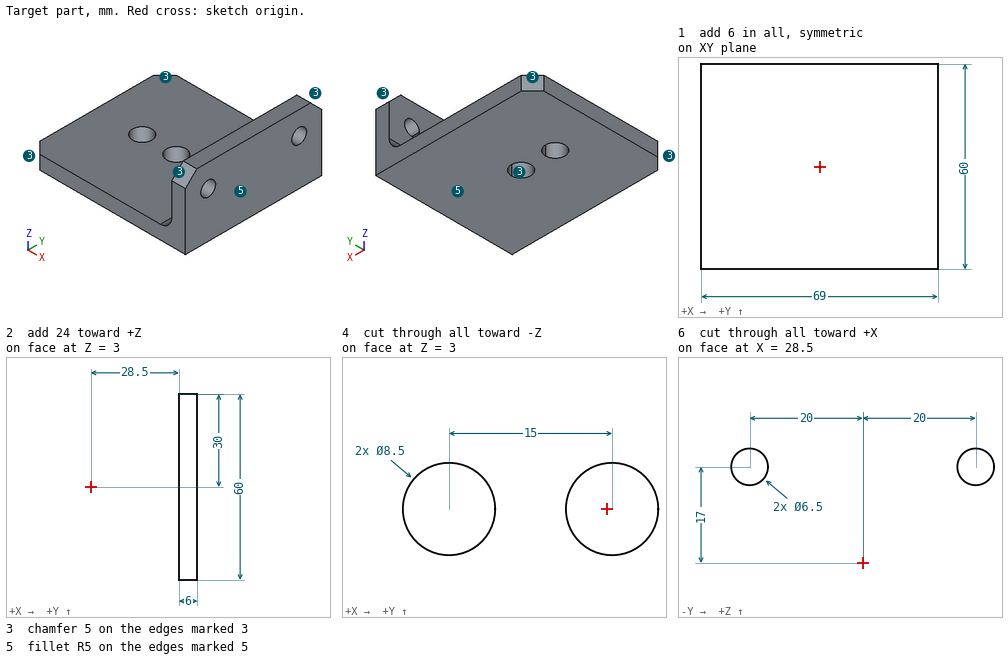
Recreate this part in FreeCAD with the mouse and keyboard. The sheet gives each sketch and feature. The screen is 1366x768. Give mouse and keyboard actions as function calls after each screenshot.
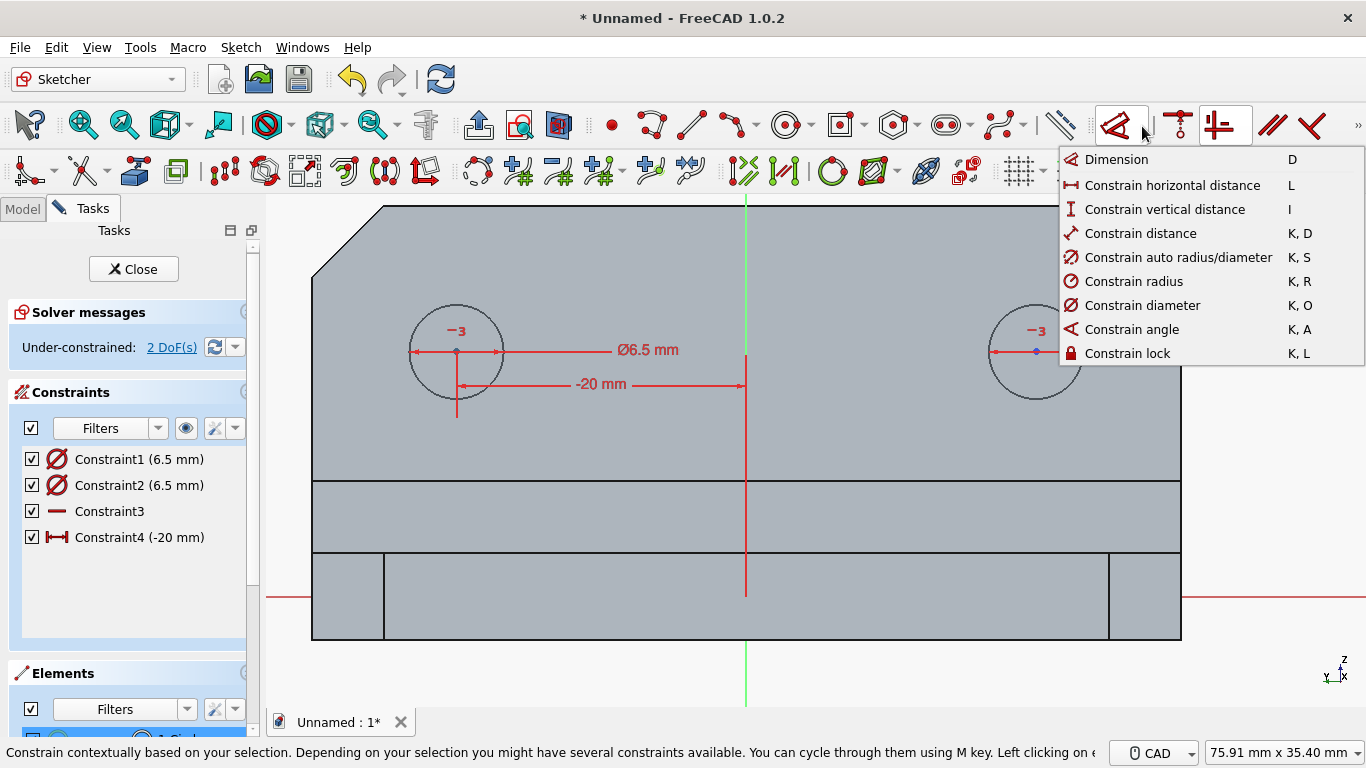
click(1212, 209)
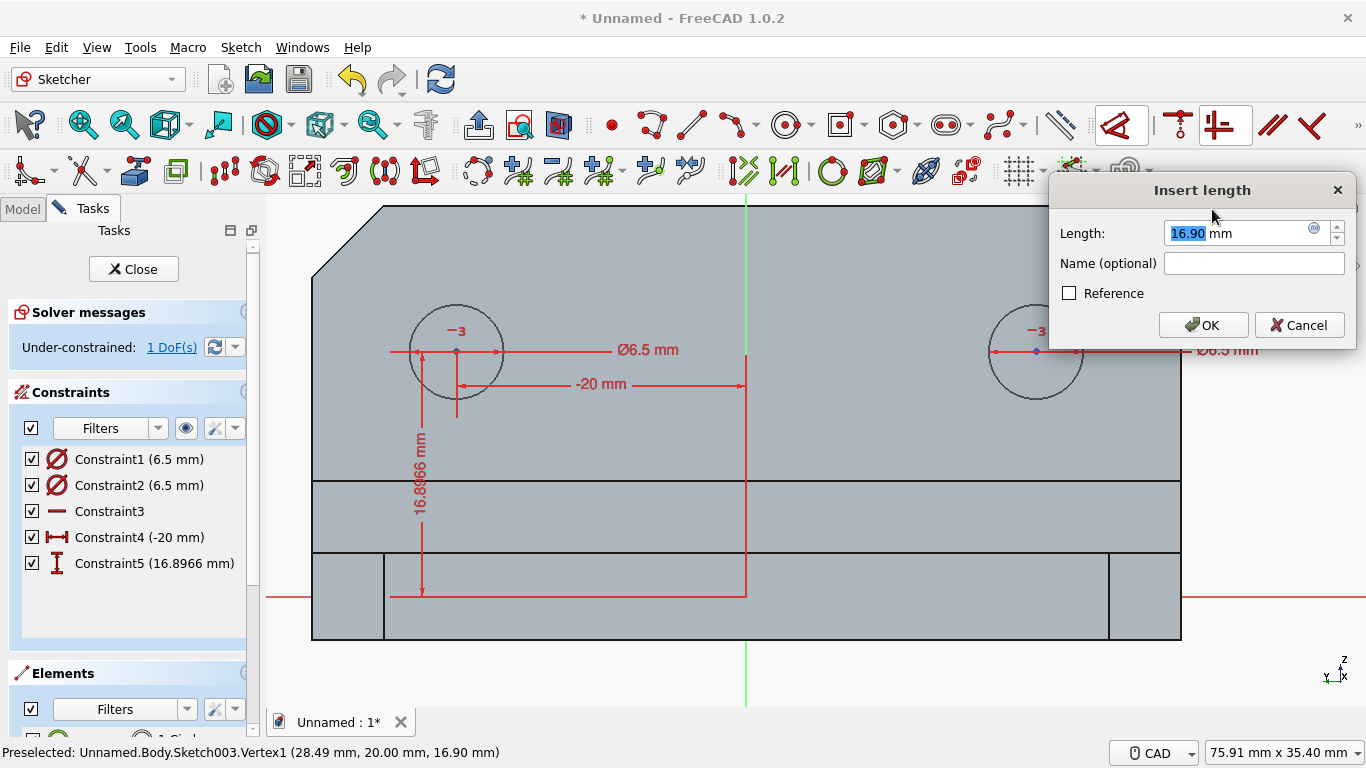
text(17)
key(Return)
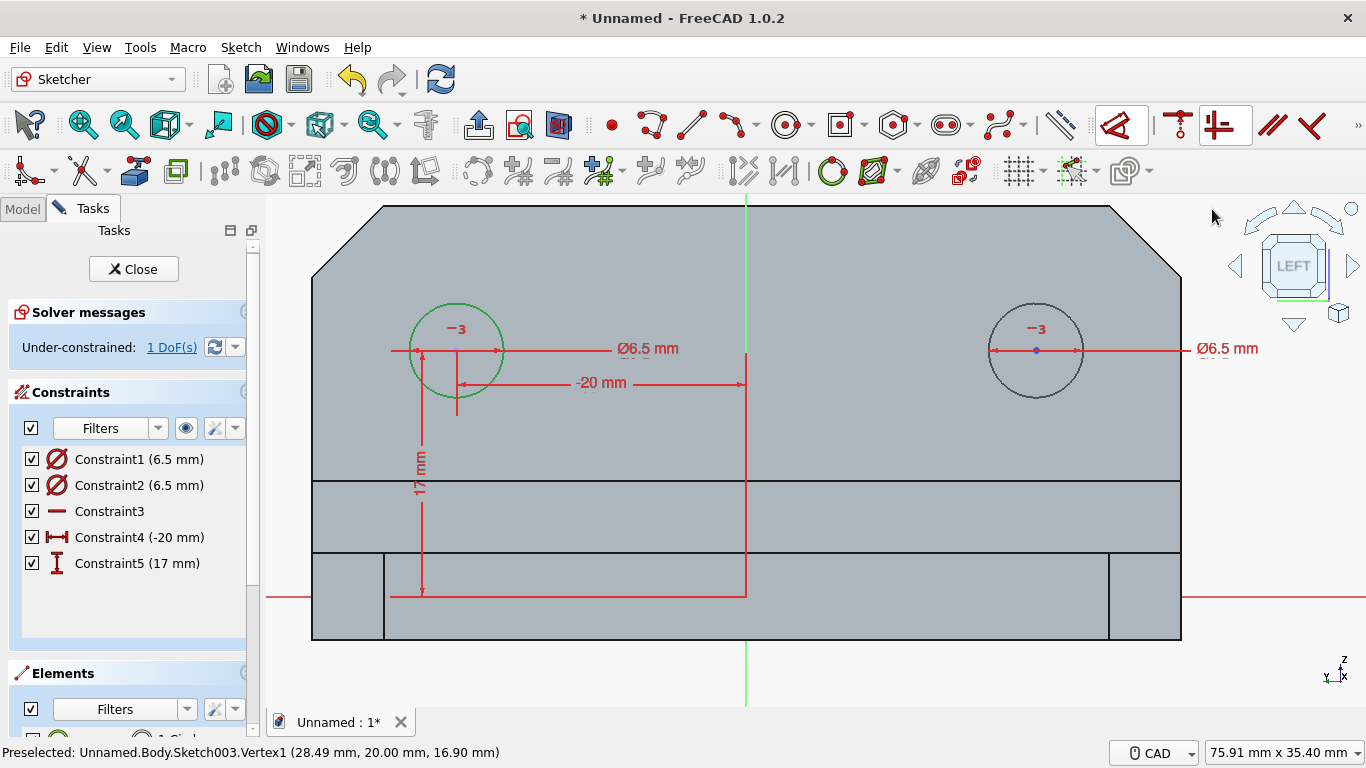
click(1036, 351)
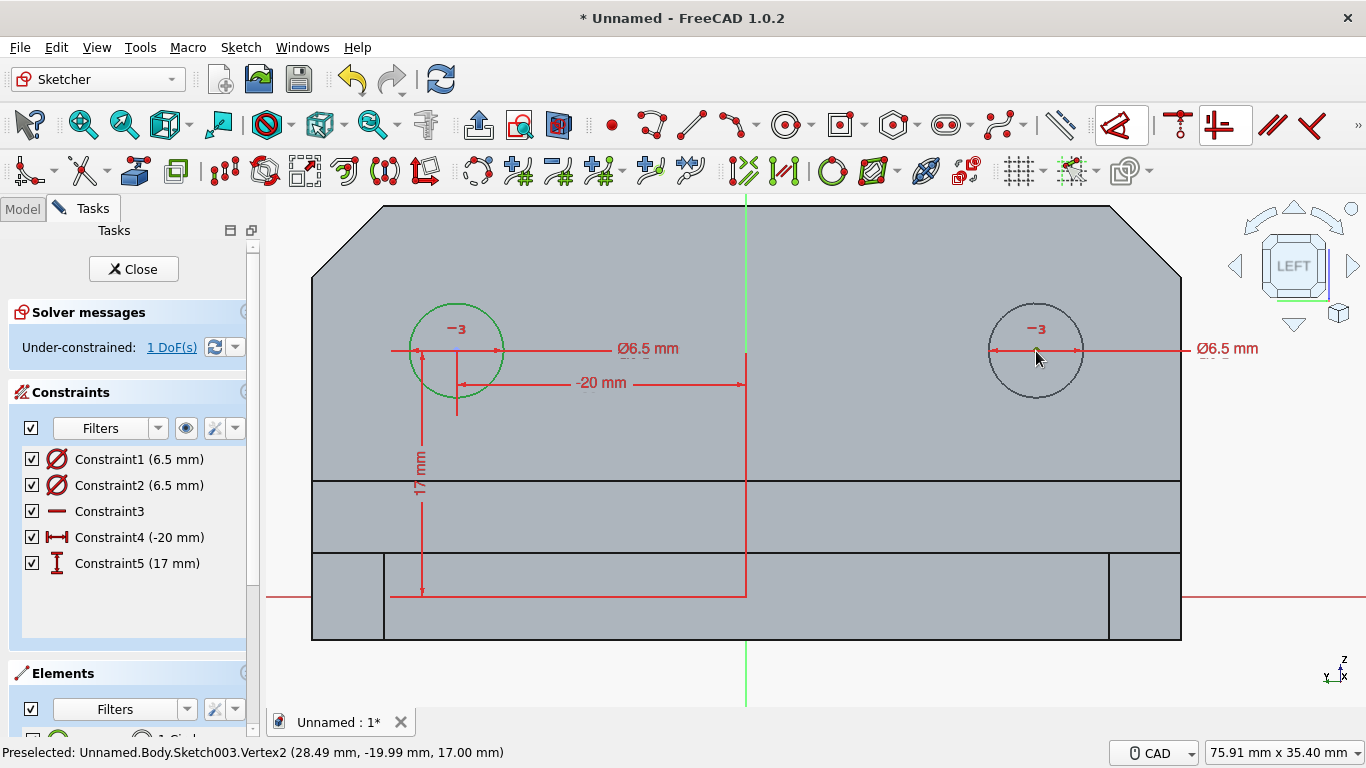
key(l)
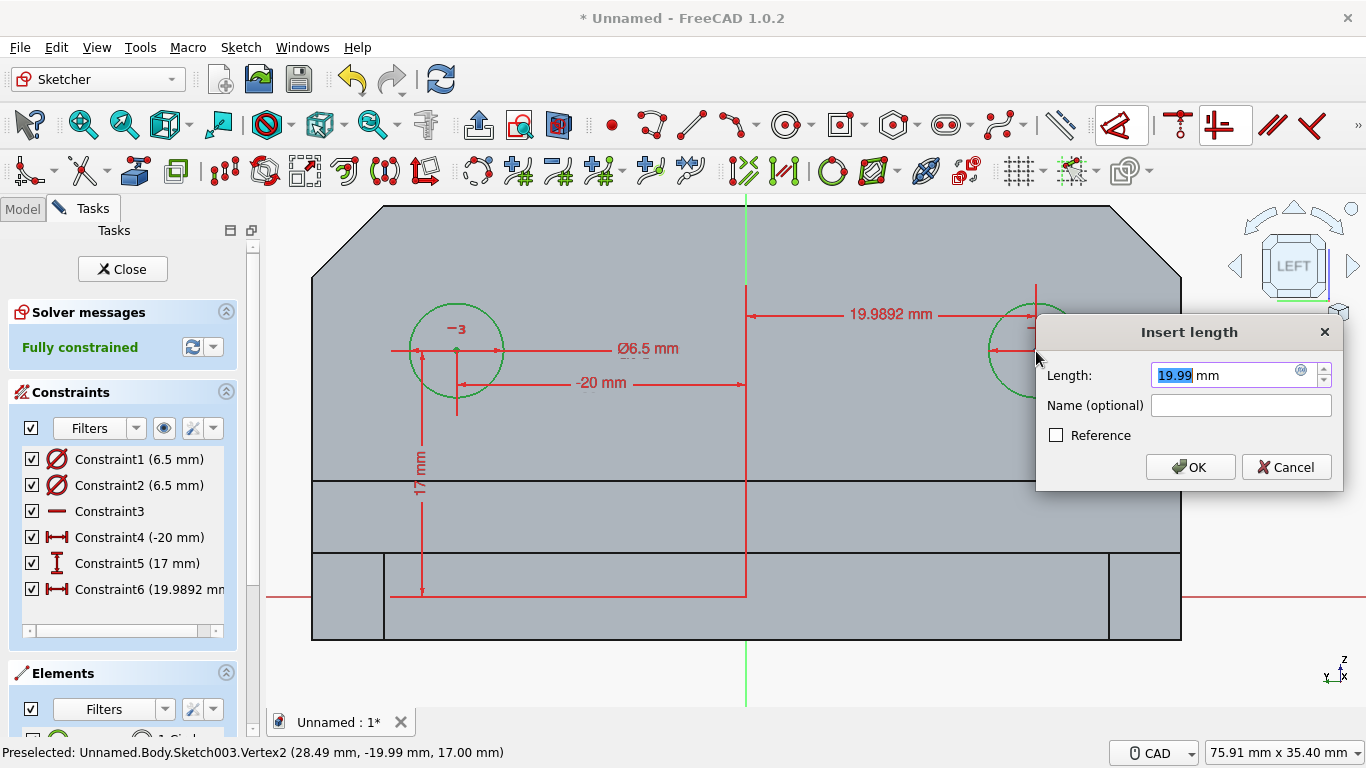
text(20)
key(Return)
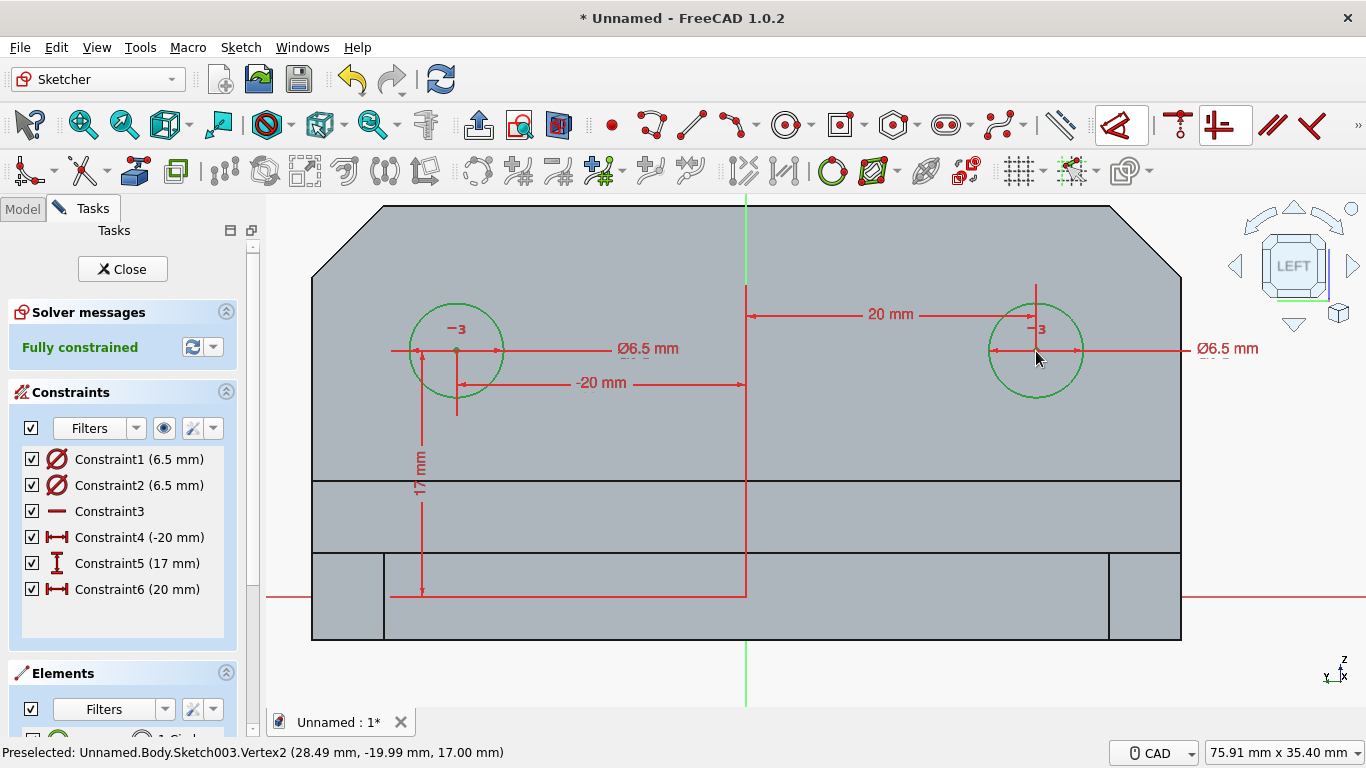
click(123, 269)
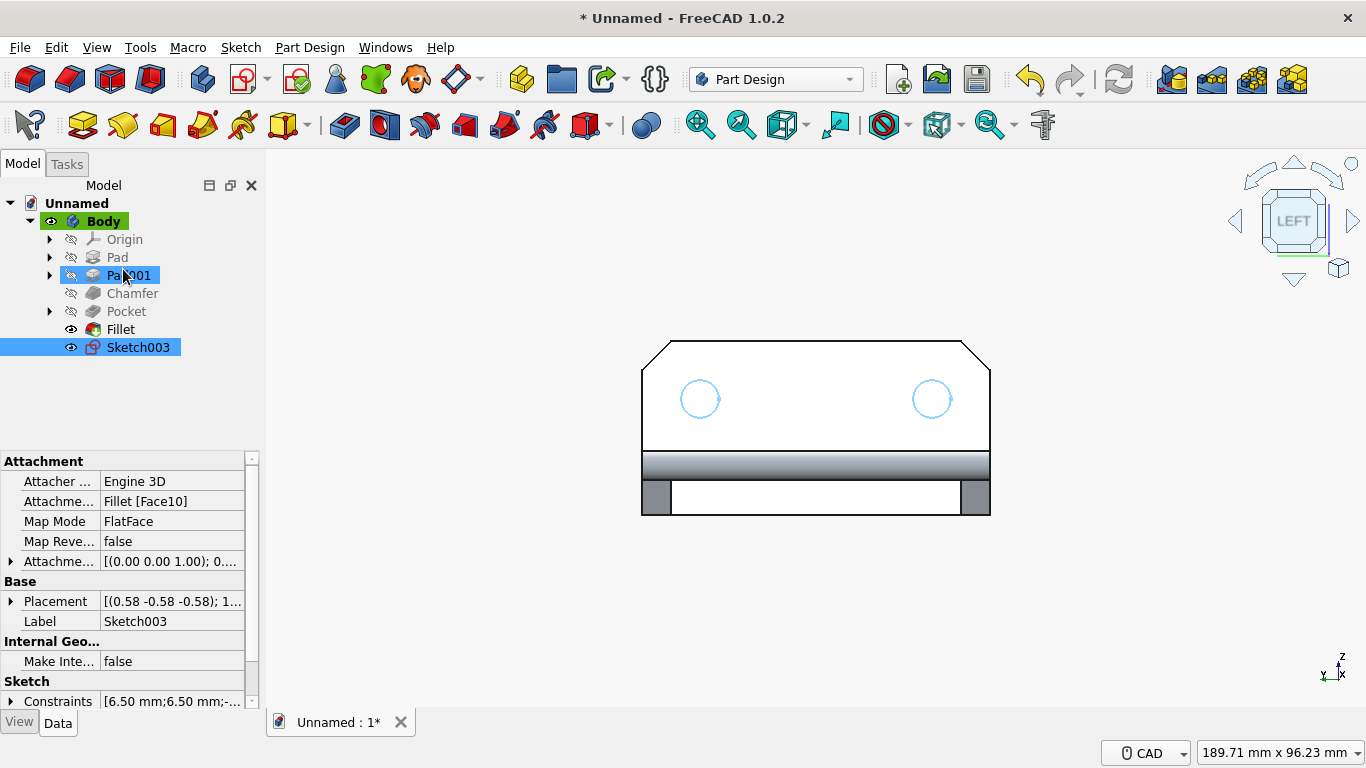
click(346, 126)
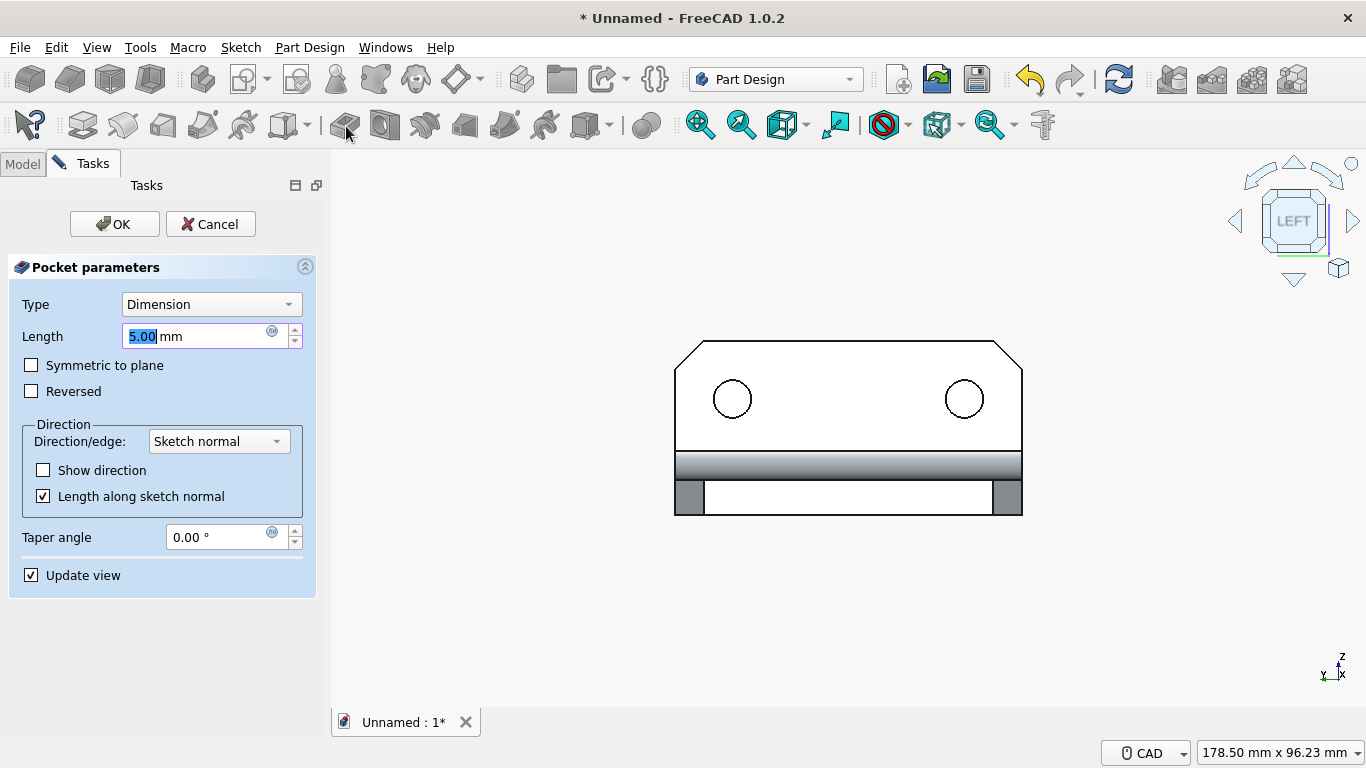
click(212, 304)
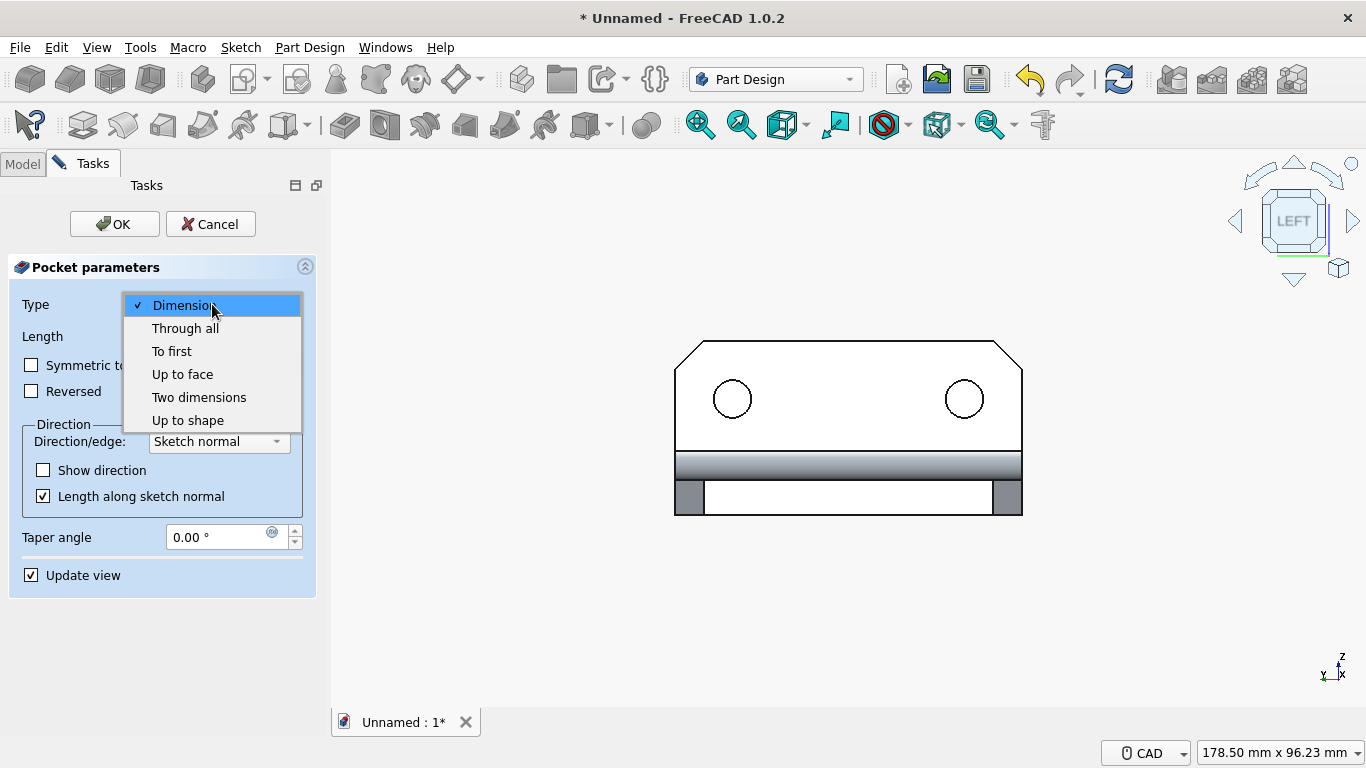
click(212, 328)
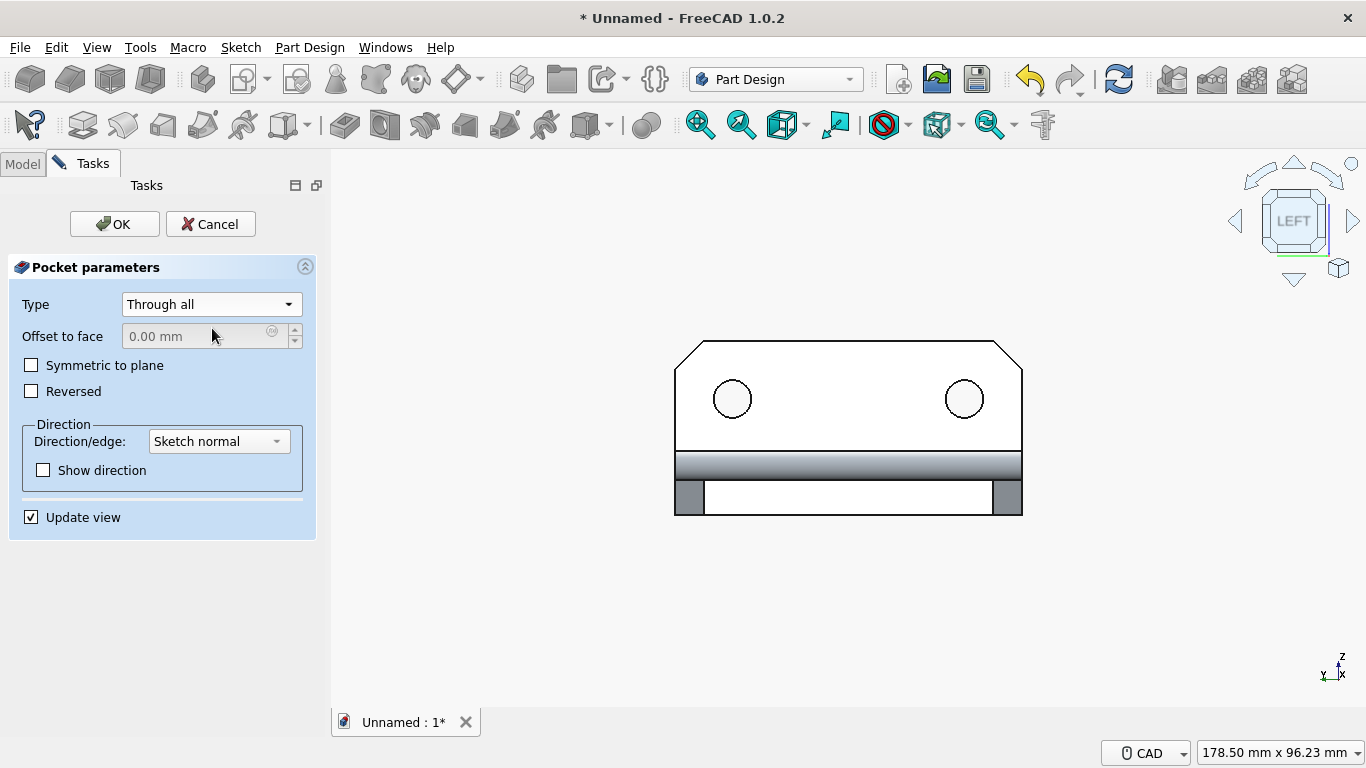
click(115, 224)